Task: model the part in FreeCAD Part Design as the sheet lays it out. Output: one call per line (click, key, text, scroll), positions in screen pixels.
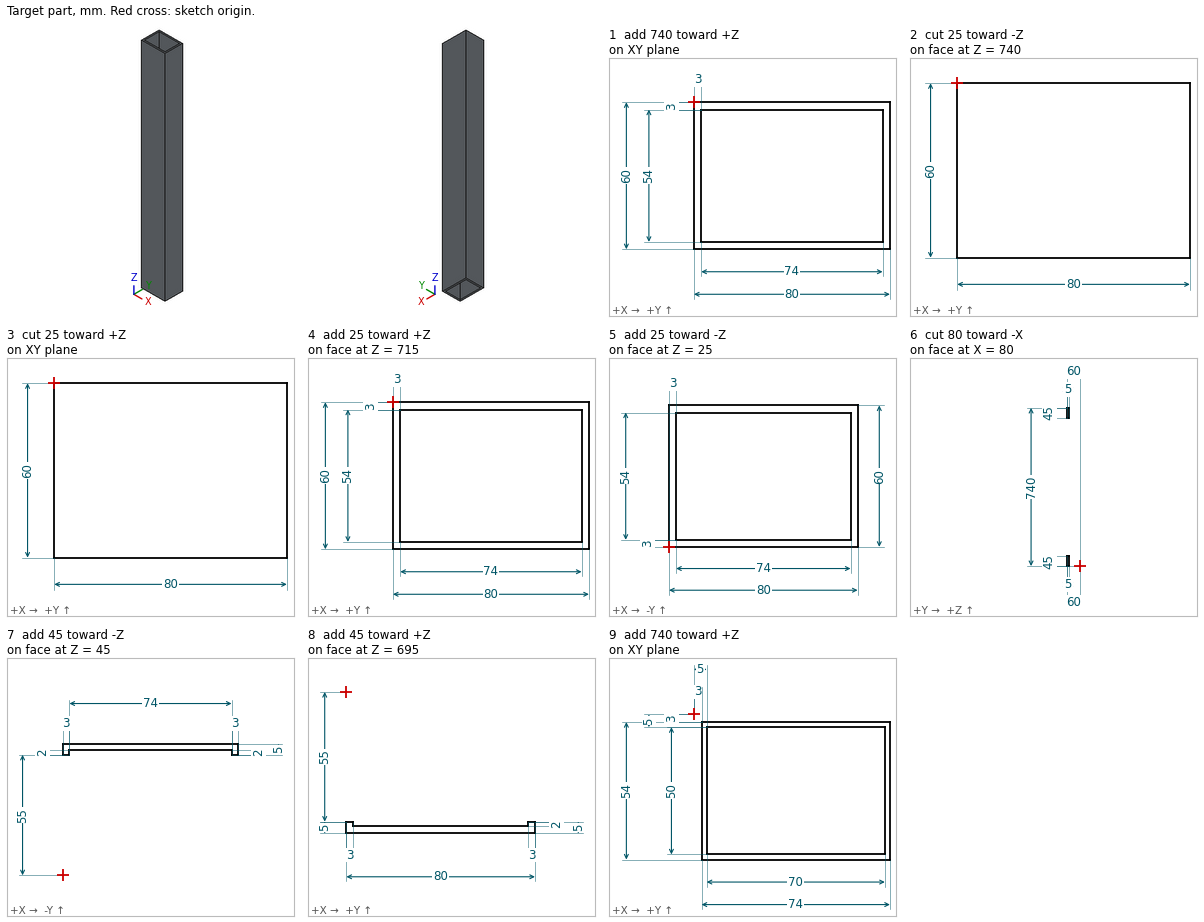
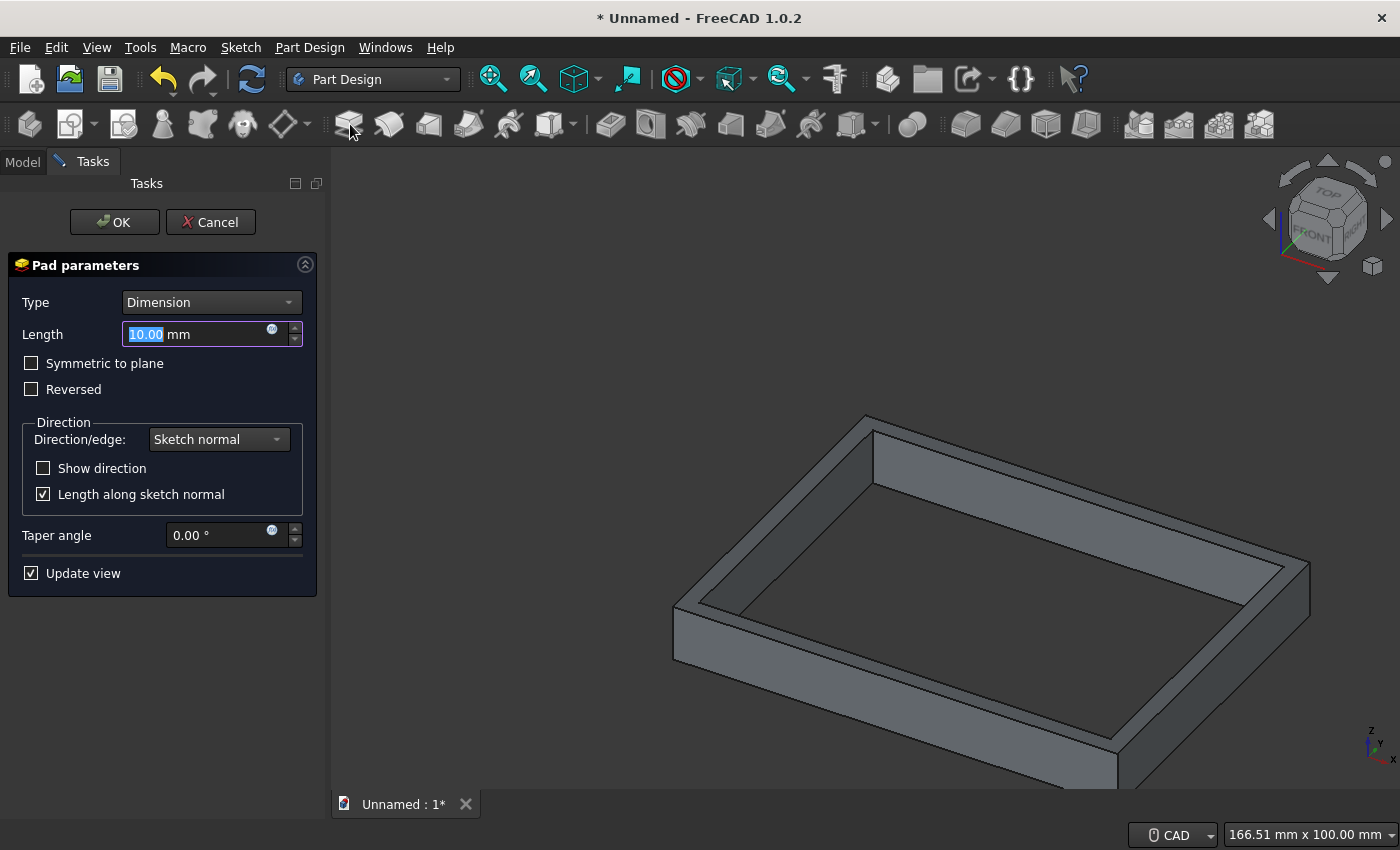
text(740)
key(Tab)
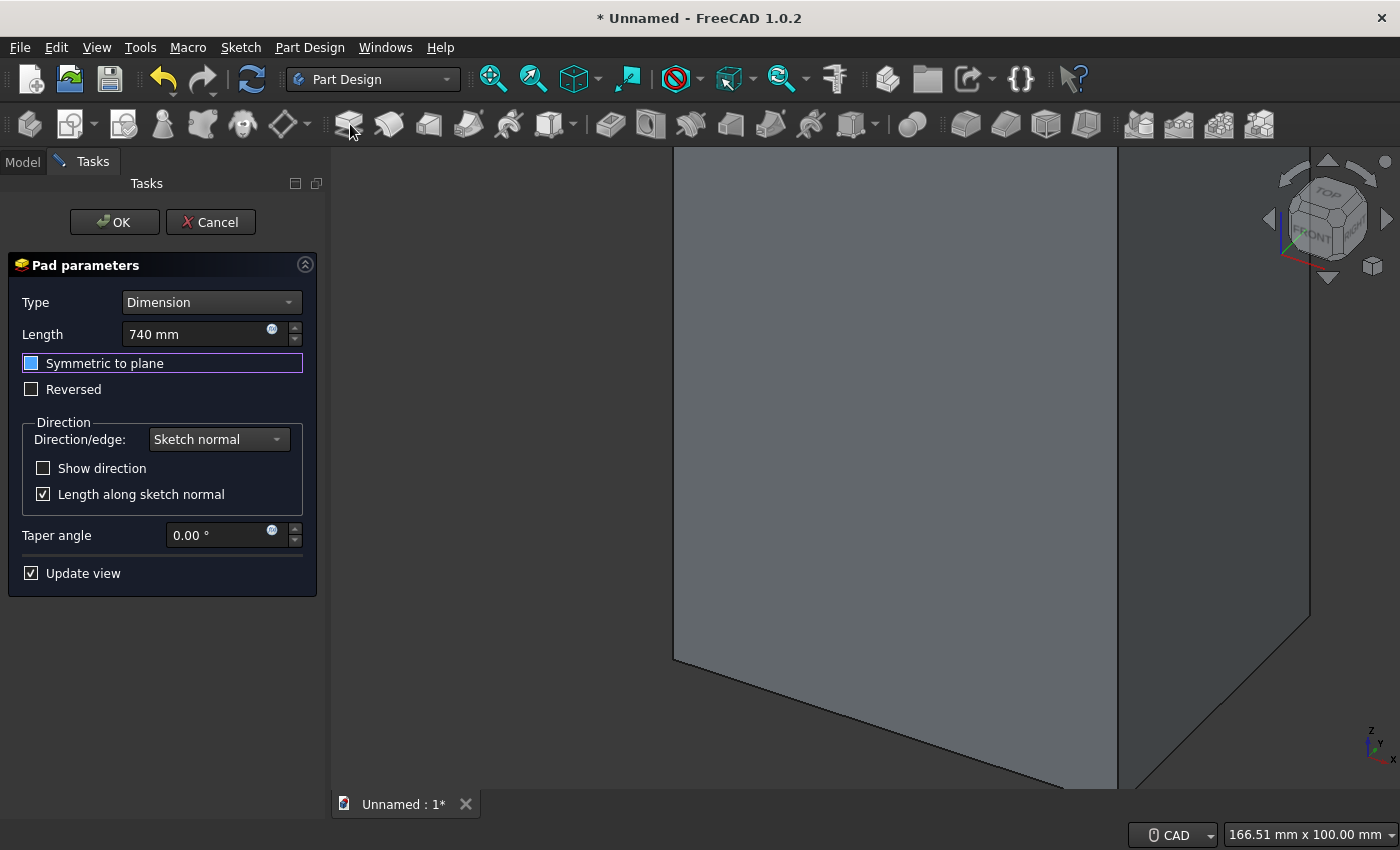
click(115, 222)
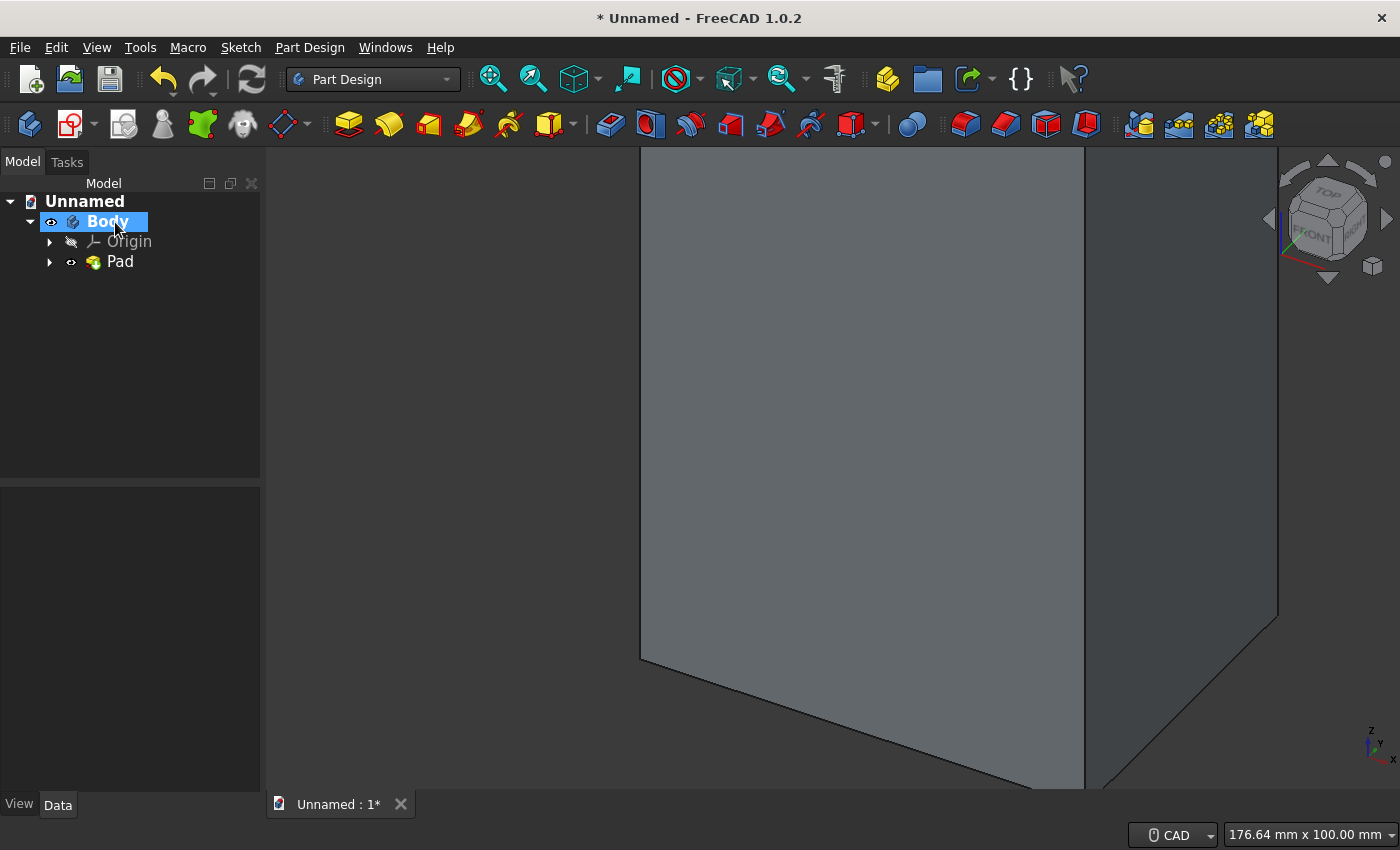
key(v)
key(f)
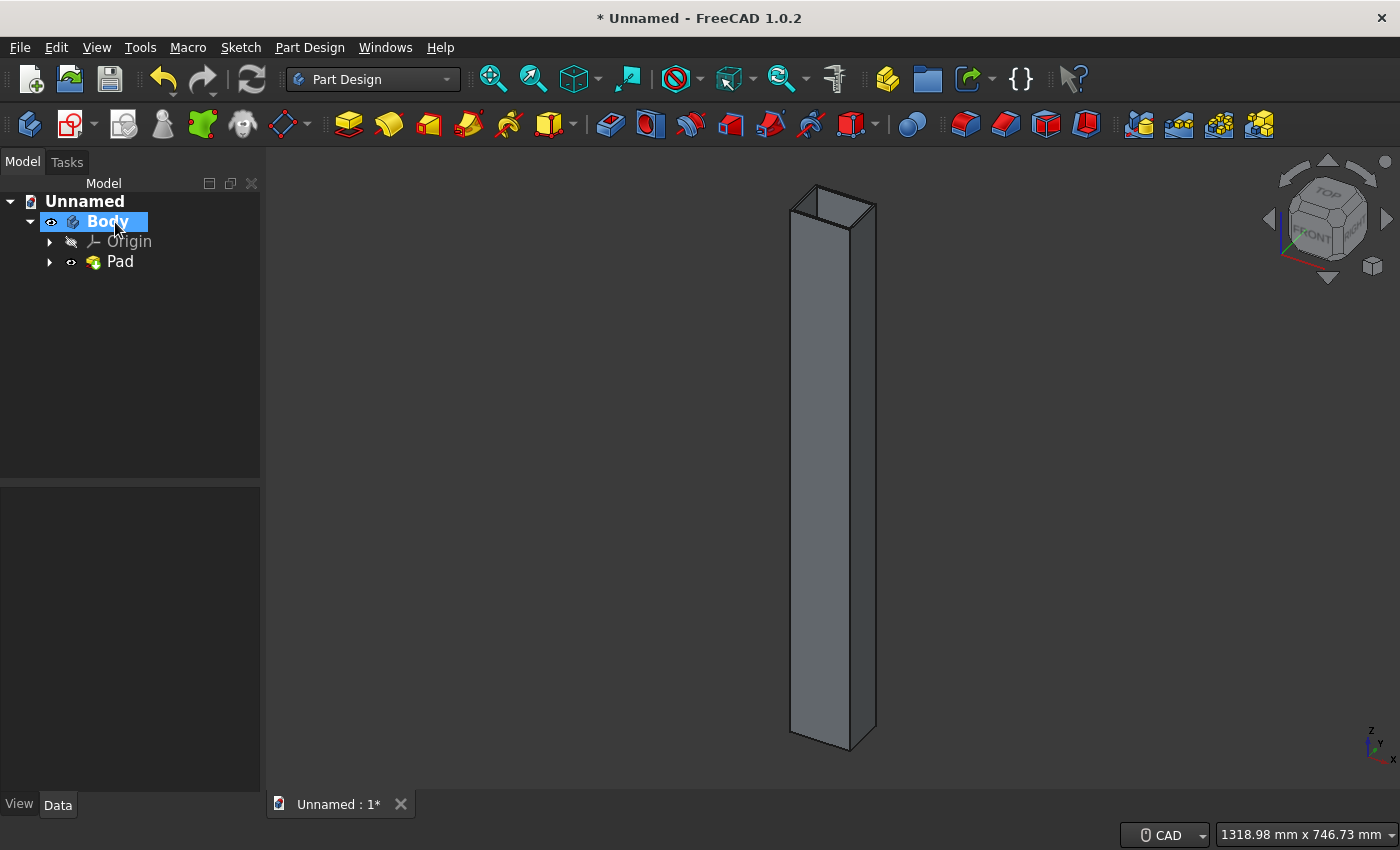
scroll(866, 212, up, 14)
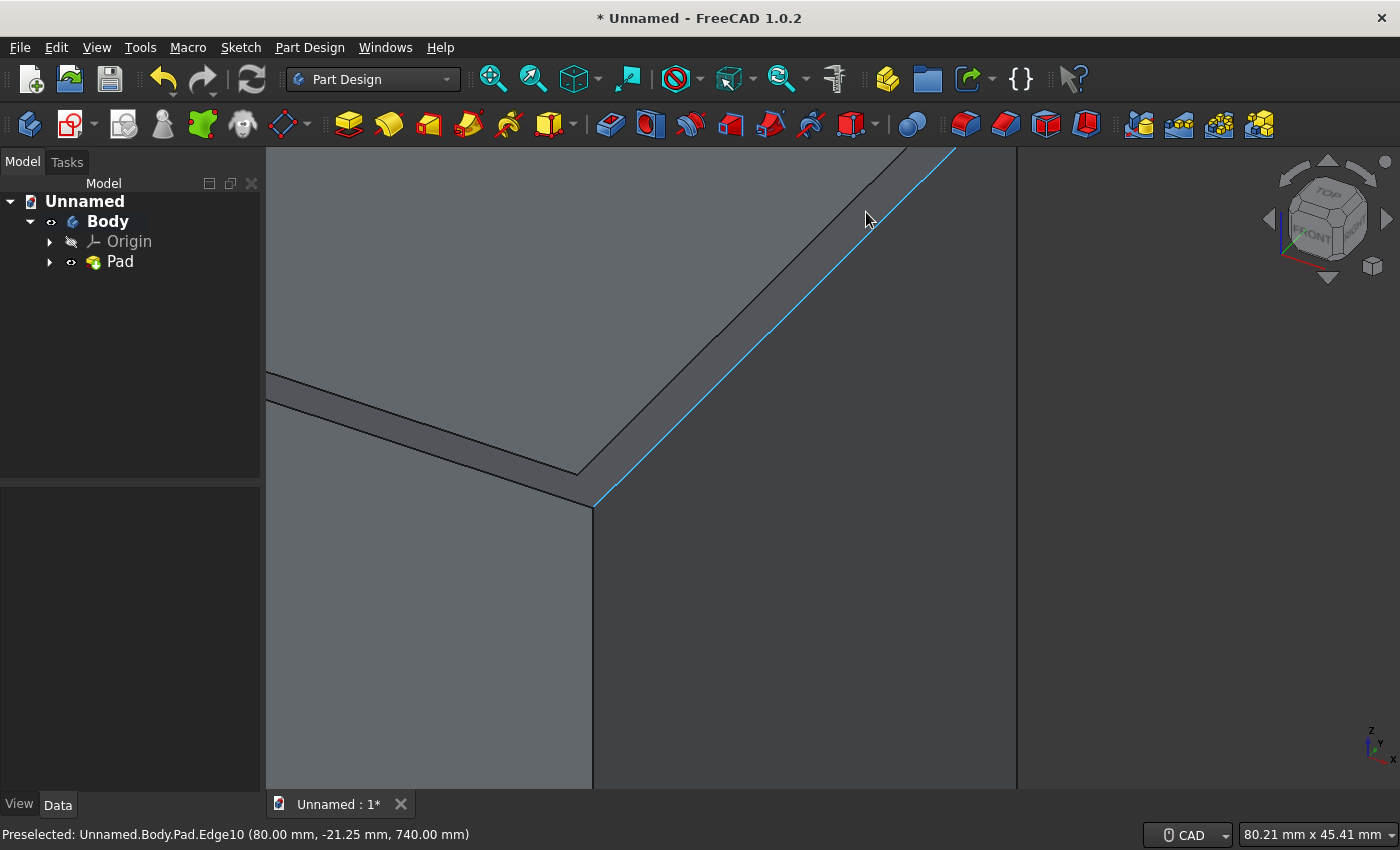
click(856, 229)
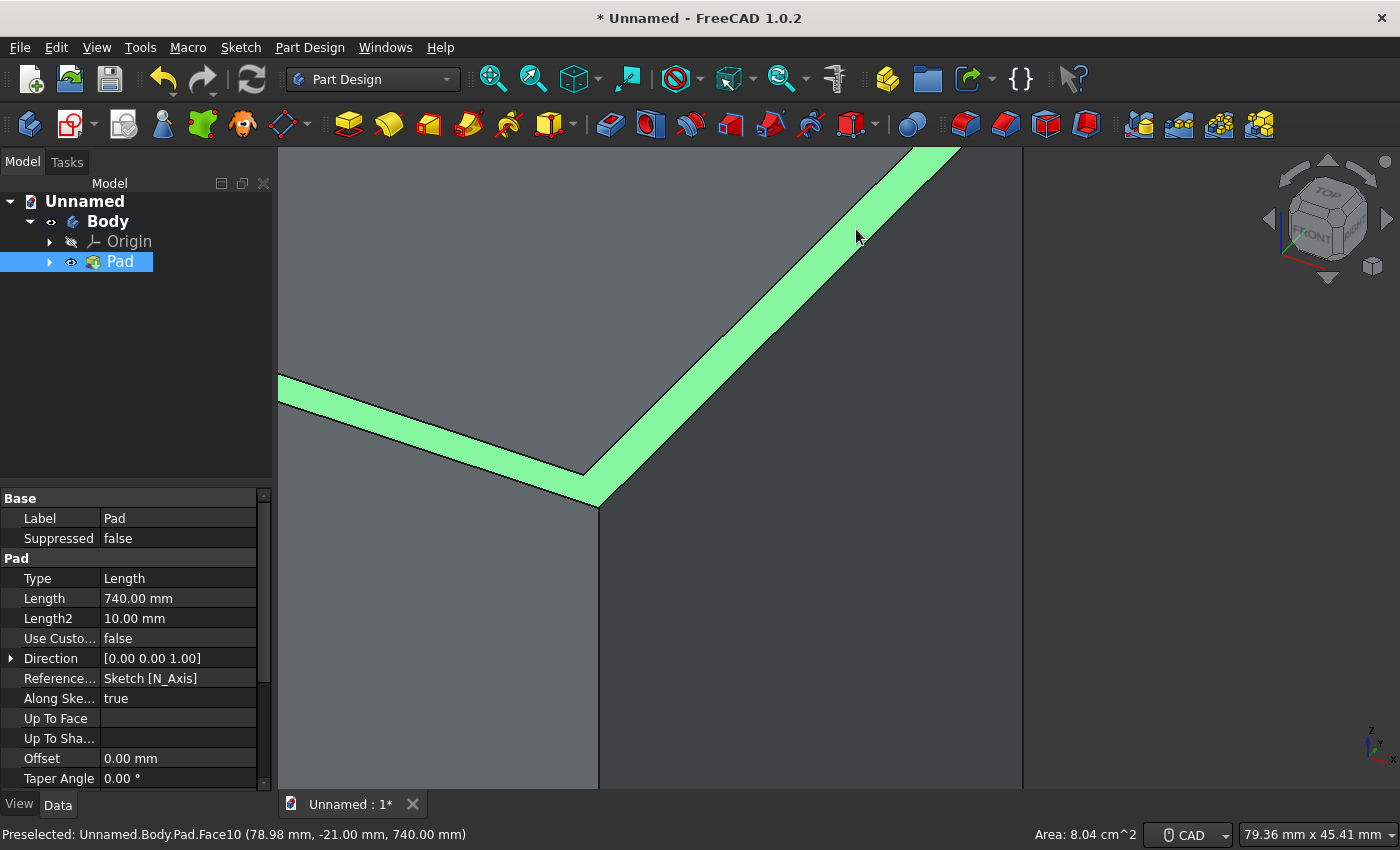
click(70, 124)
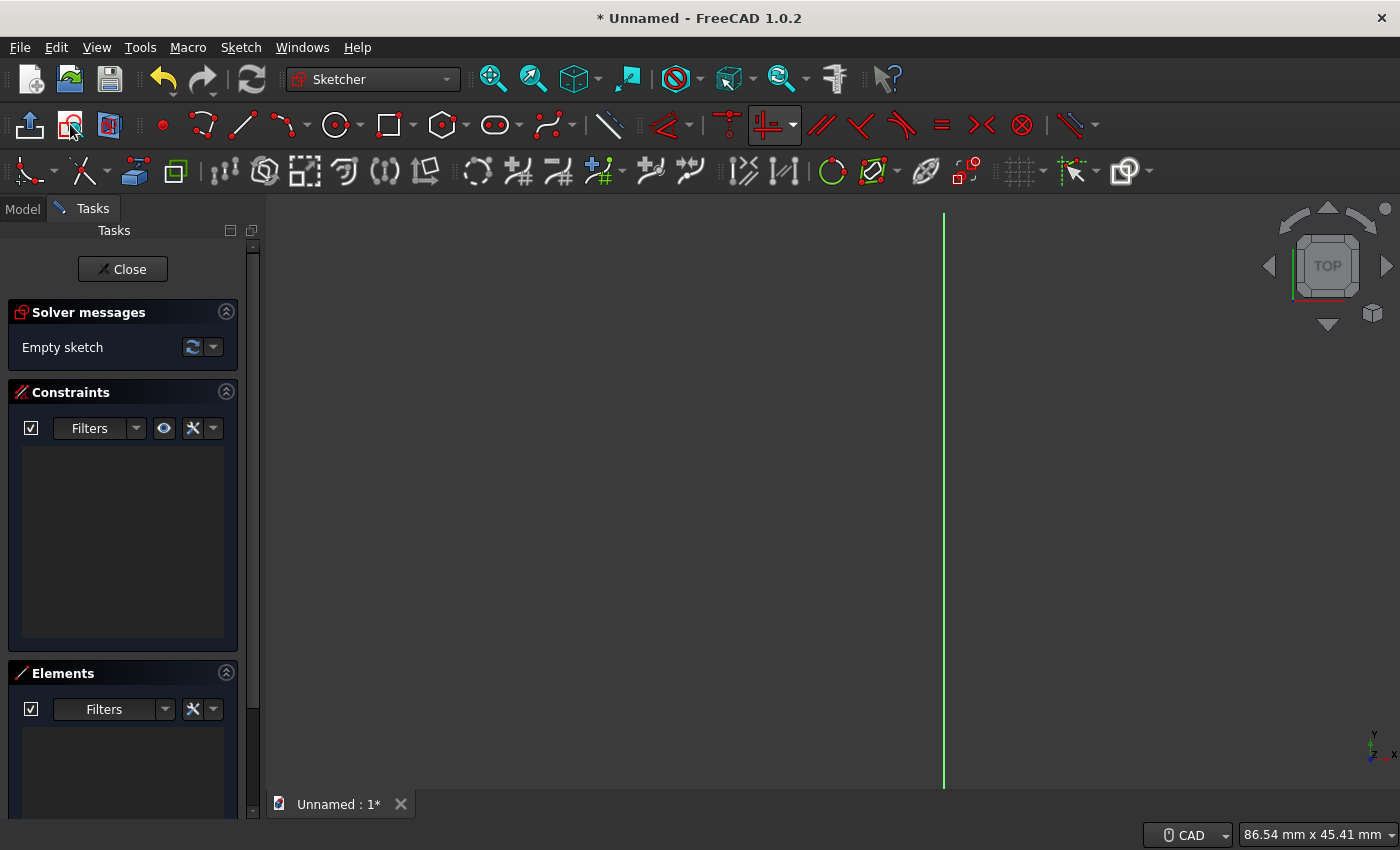
scroll(764, 492, down, 5)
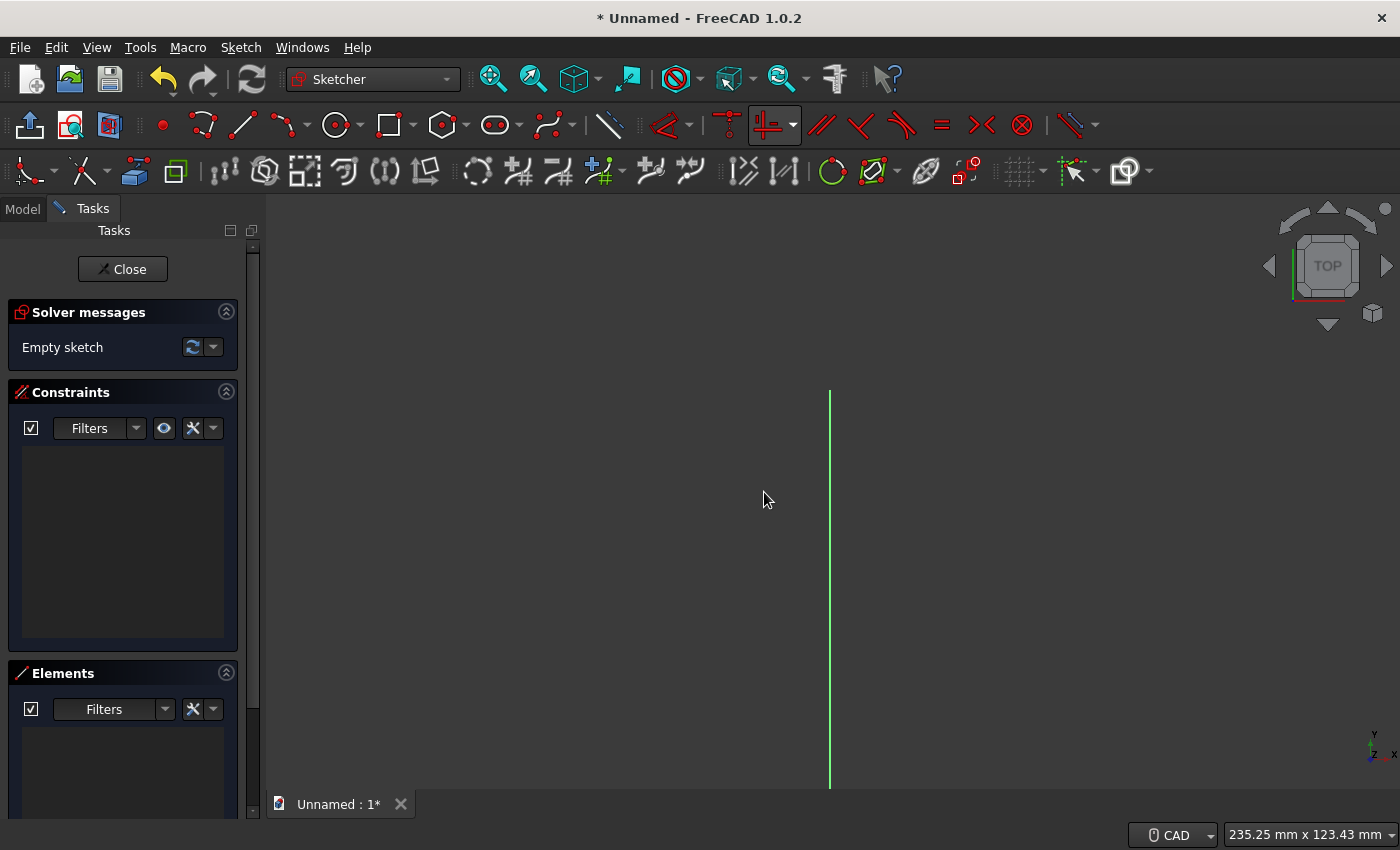
scroll(764, 492, down, 5)